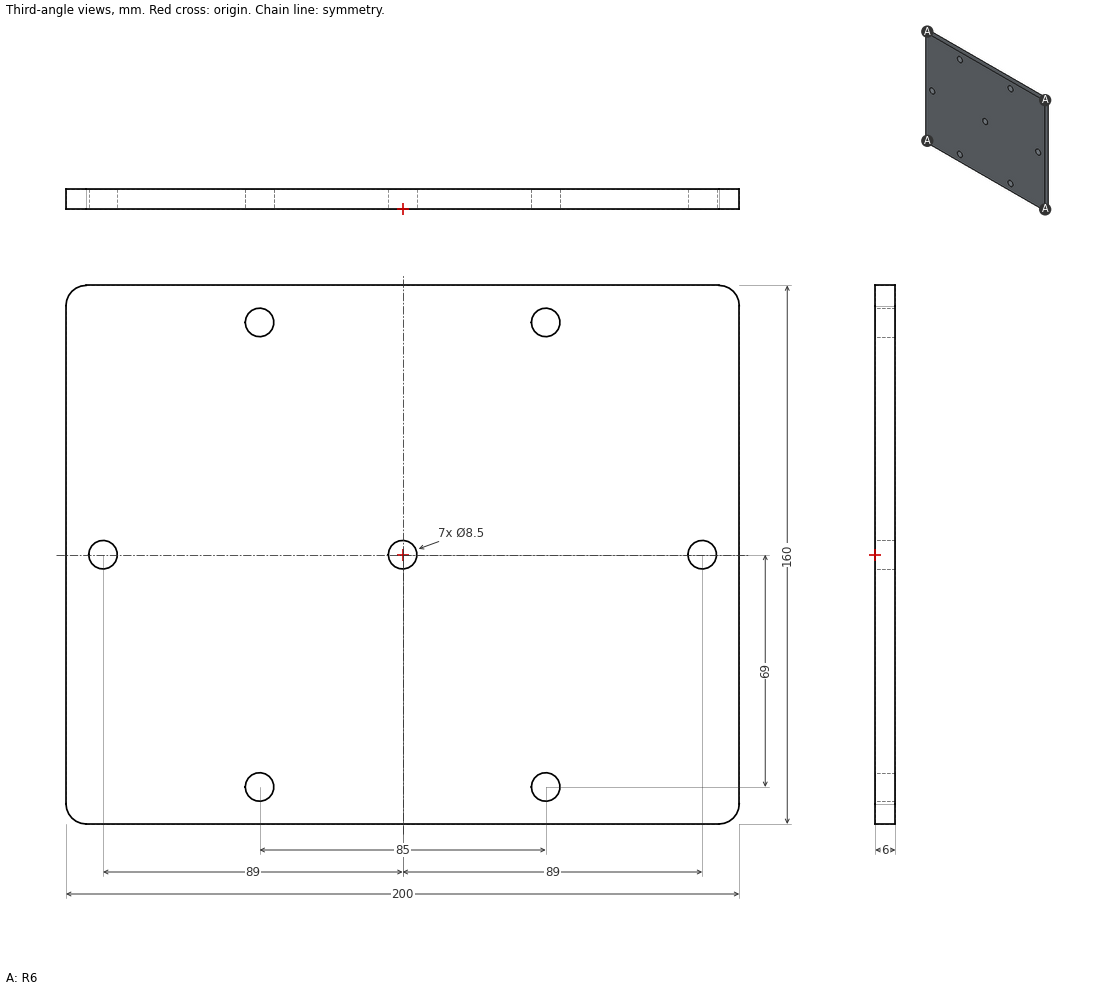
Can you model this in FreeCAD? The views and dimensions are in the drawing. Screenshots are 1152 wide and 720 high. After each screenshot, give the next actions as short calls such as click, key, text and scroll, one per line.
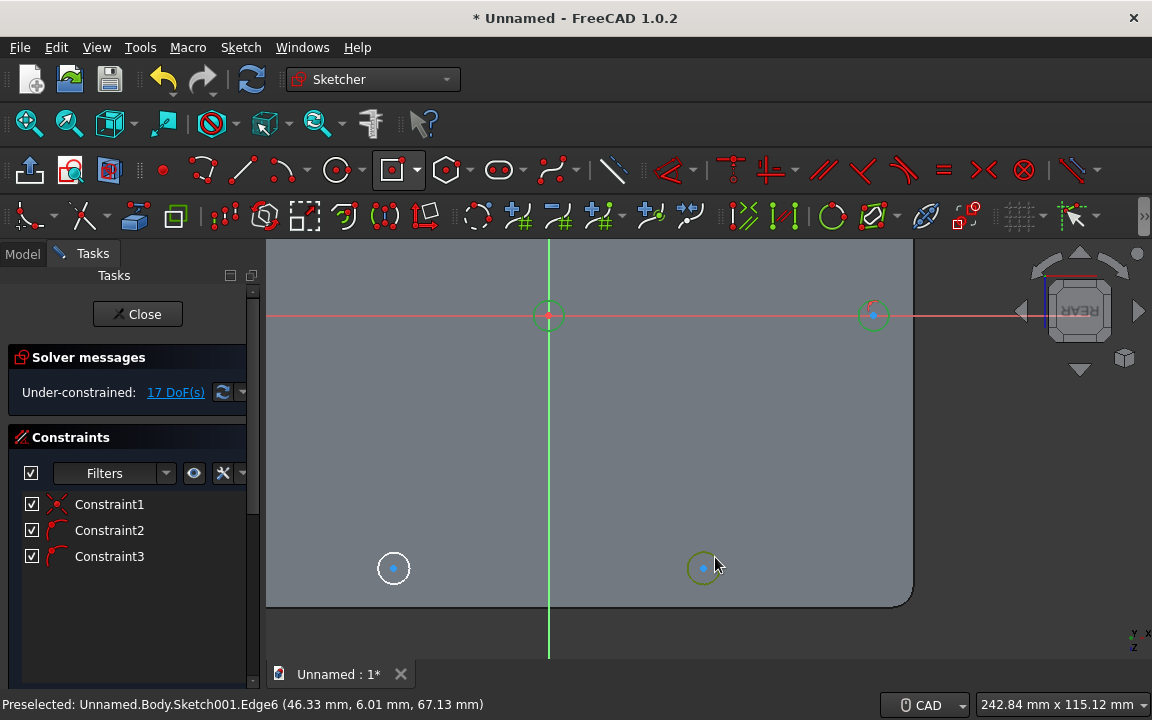
click(405, 557)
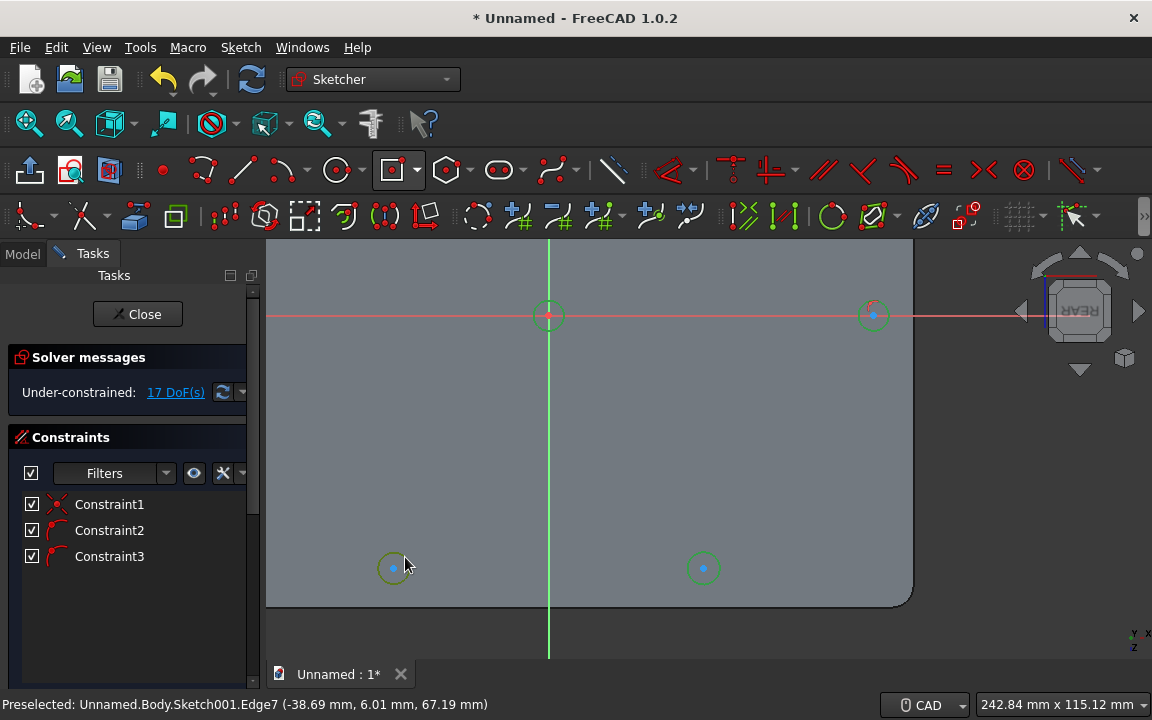
click(944, 170)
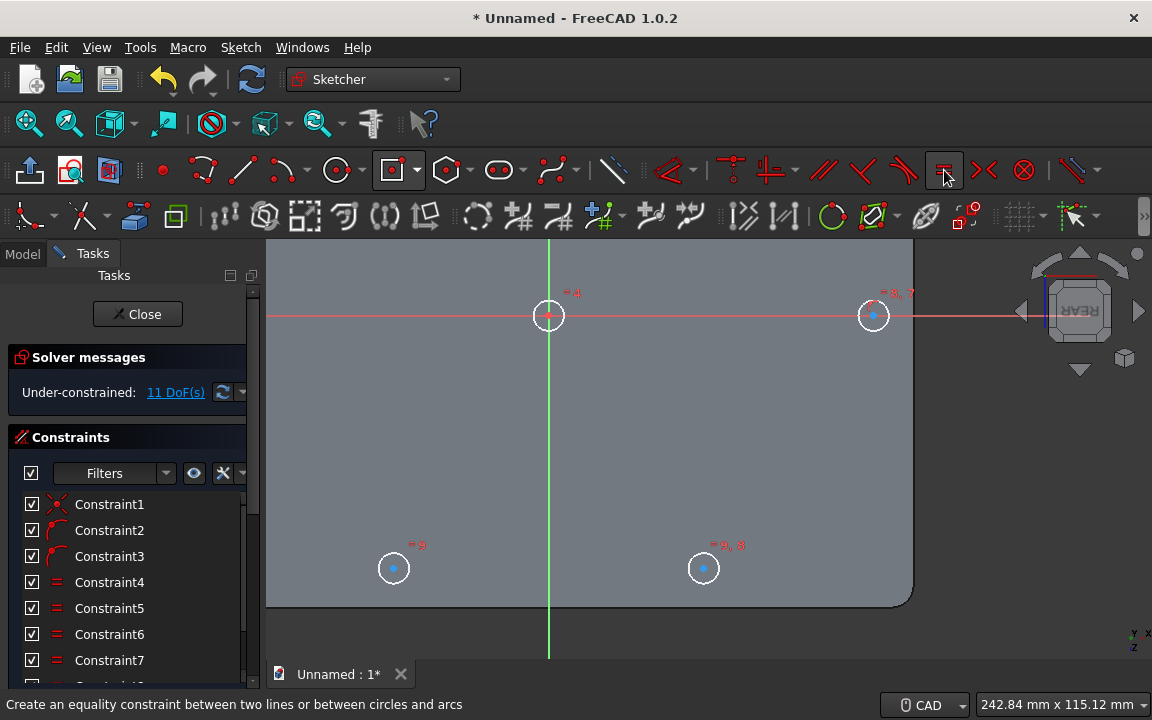
scroll(715, 558, down, 4)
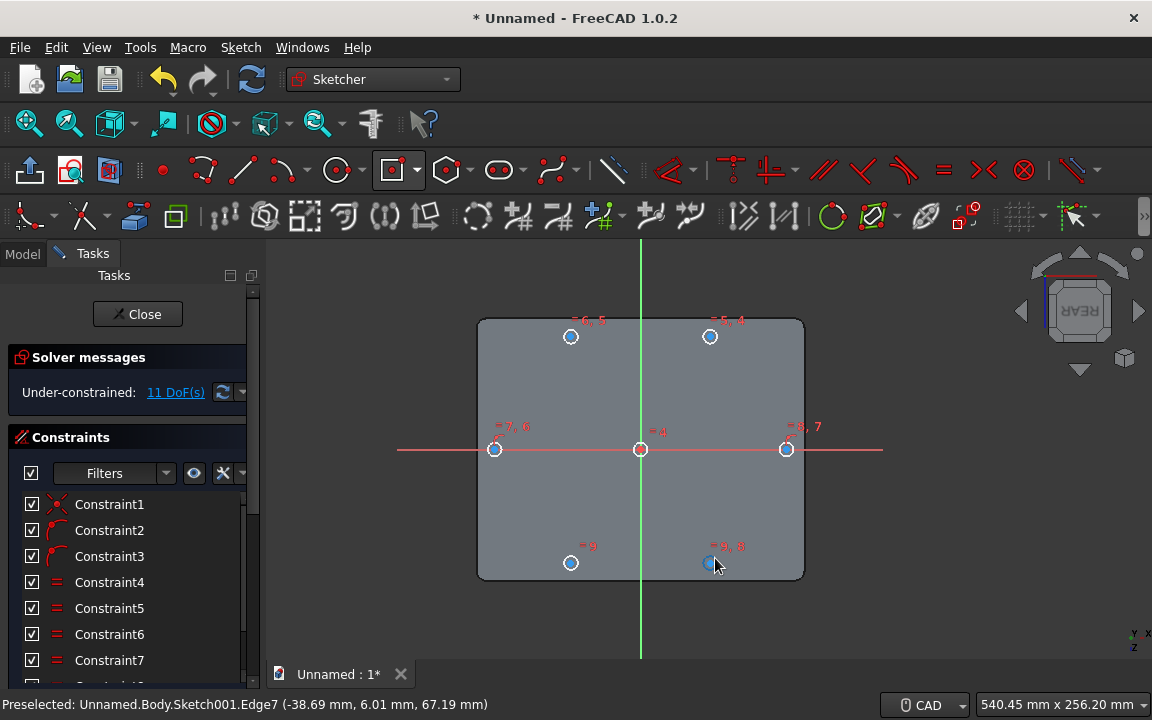
click(710, 337)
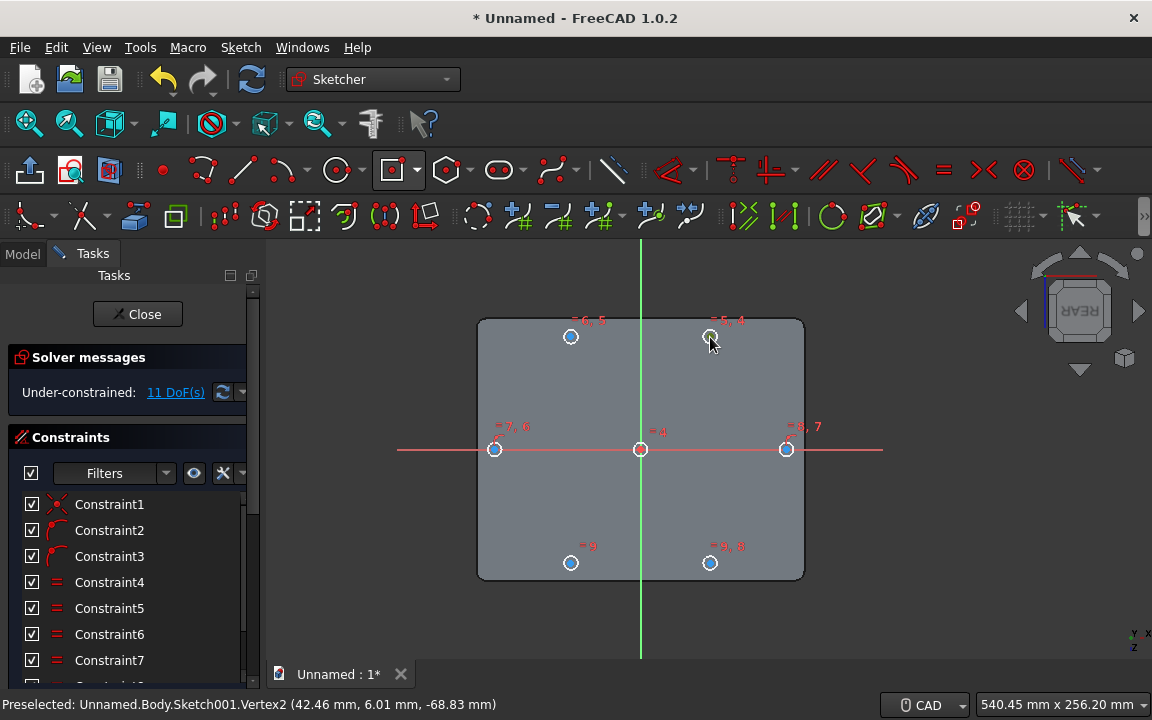
click(571, 337)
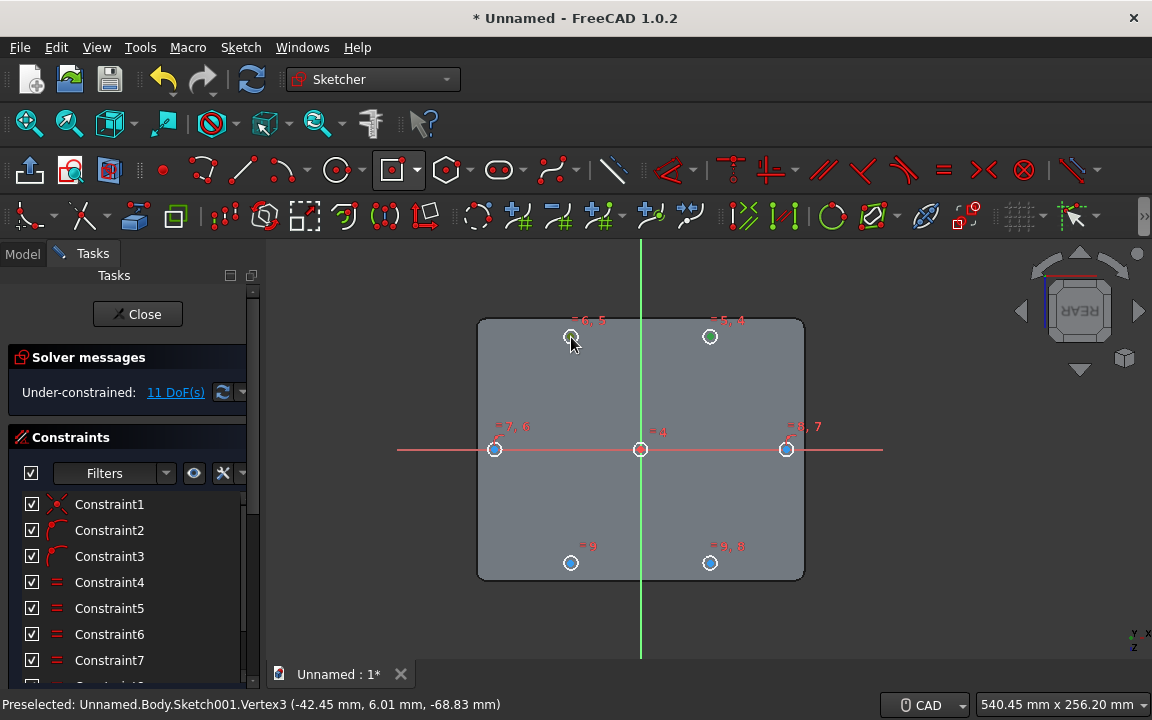
click(641, 605)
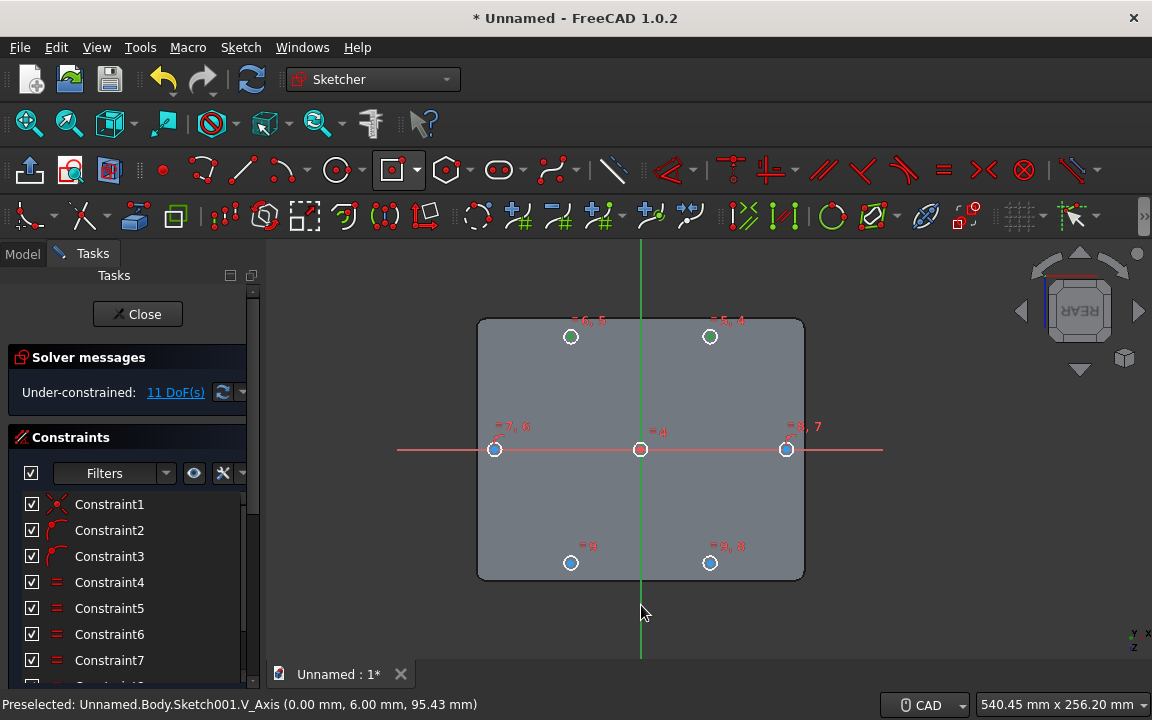
click(984, 170)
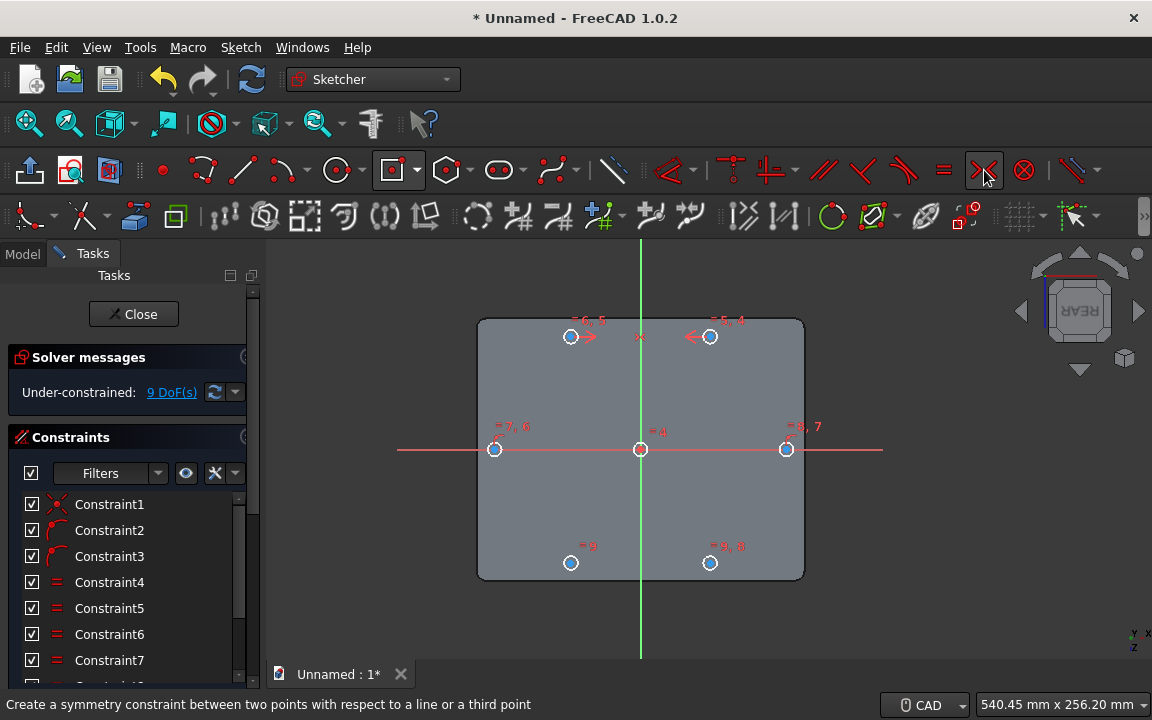
click(710, 337)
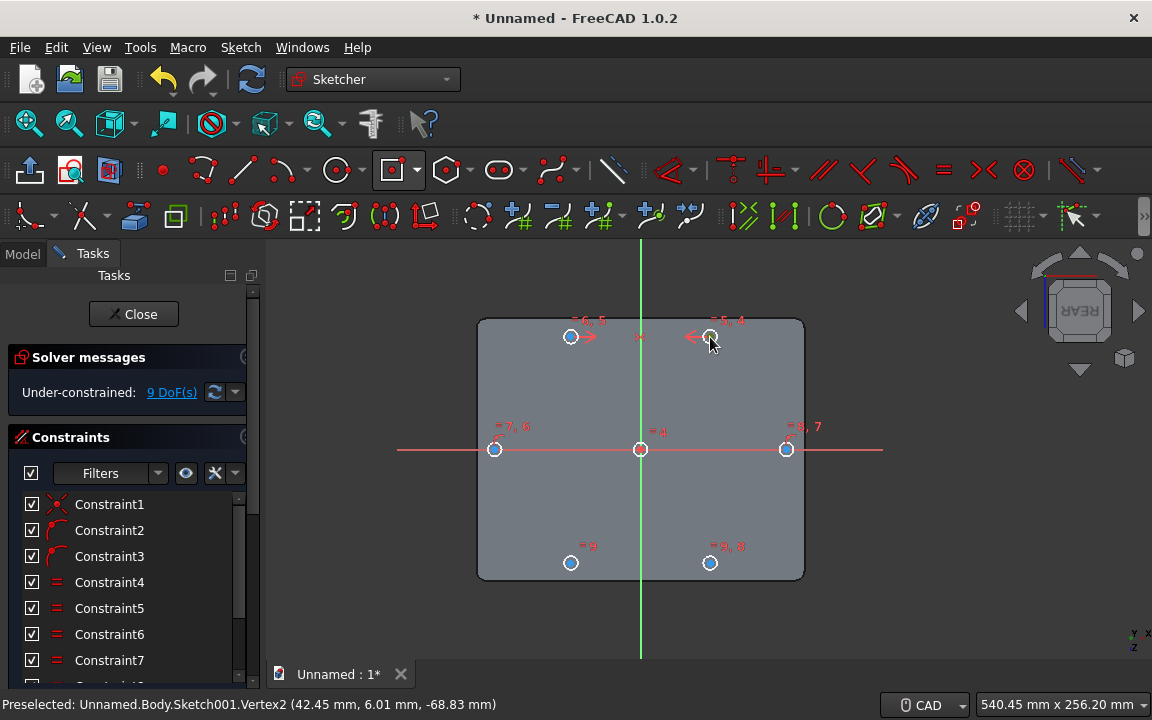
click(710, 563)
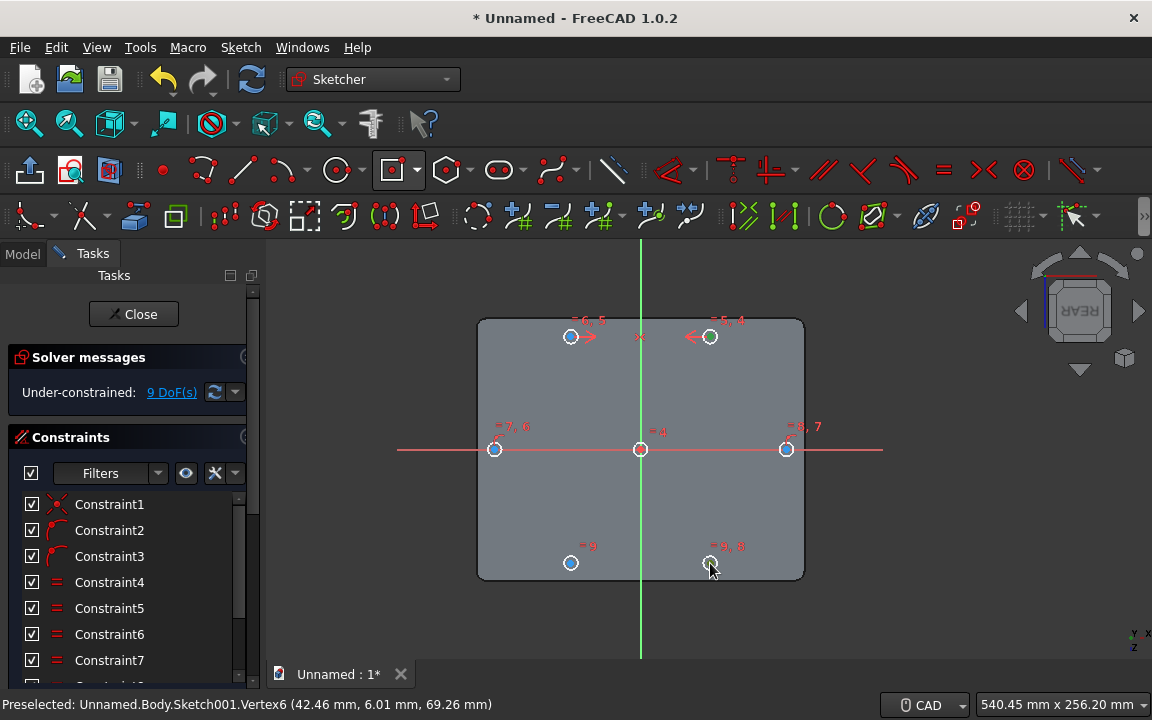
click(393, 450)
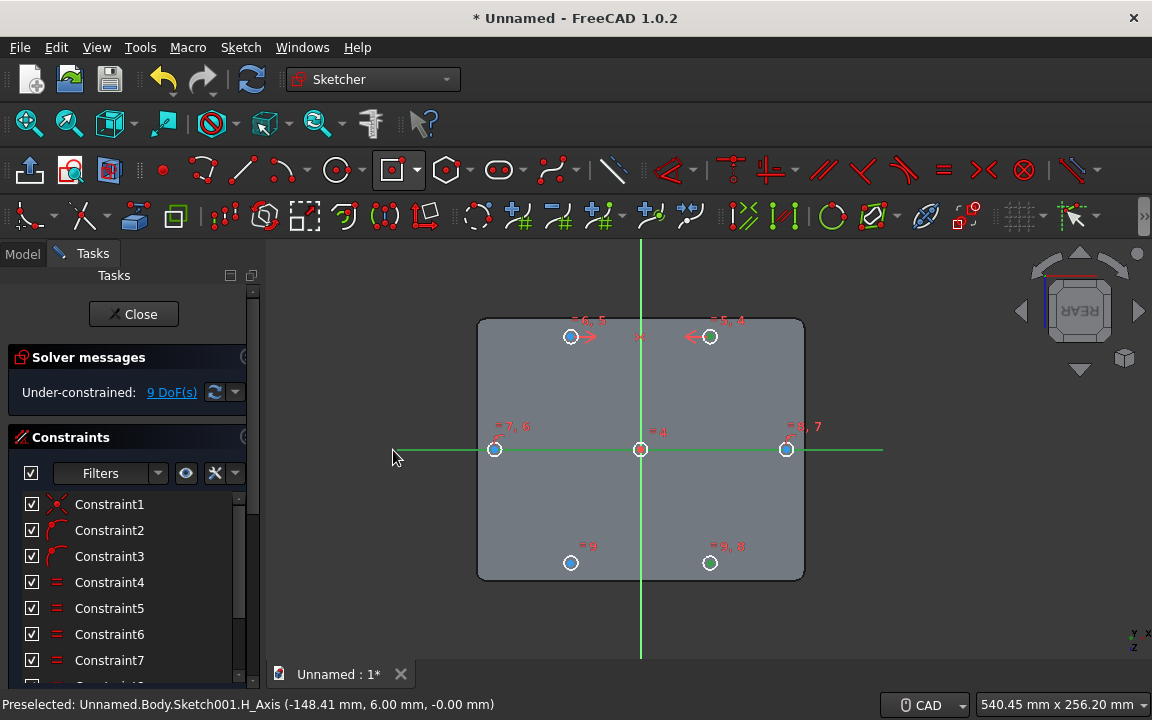
click(984, 170)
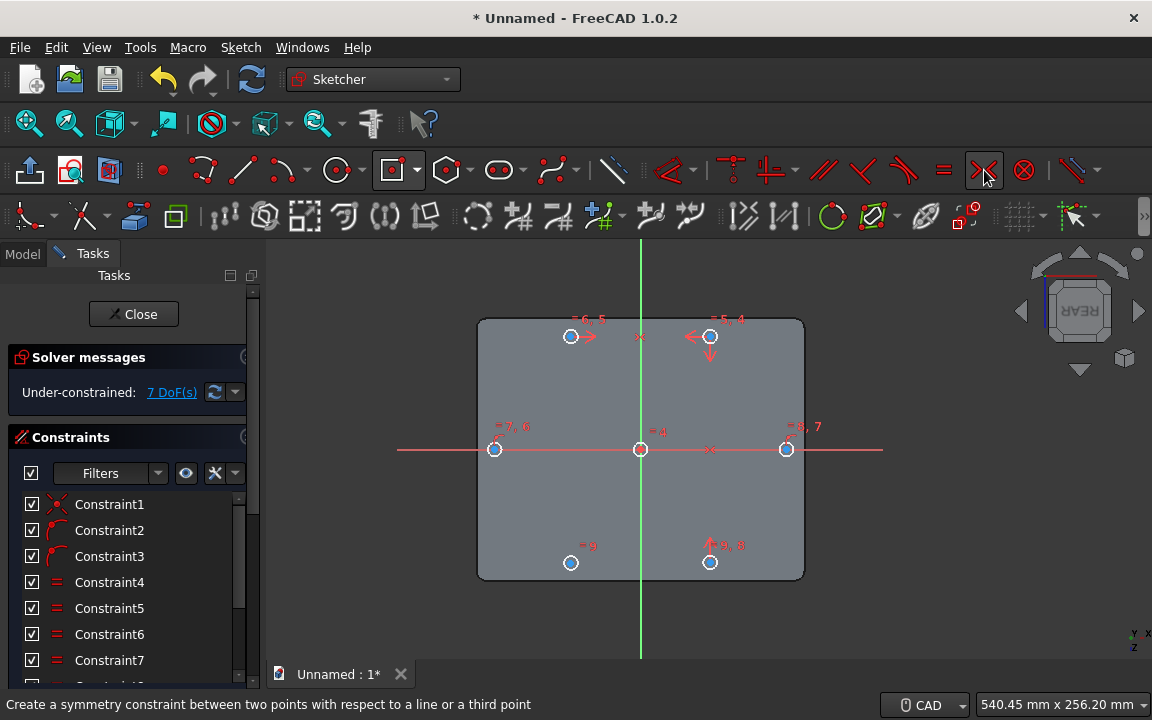
click(571, 337)